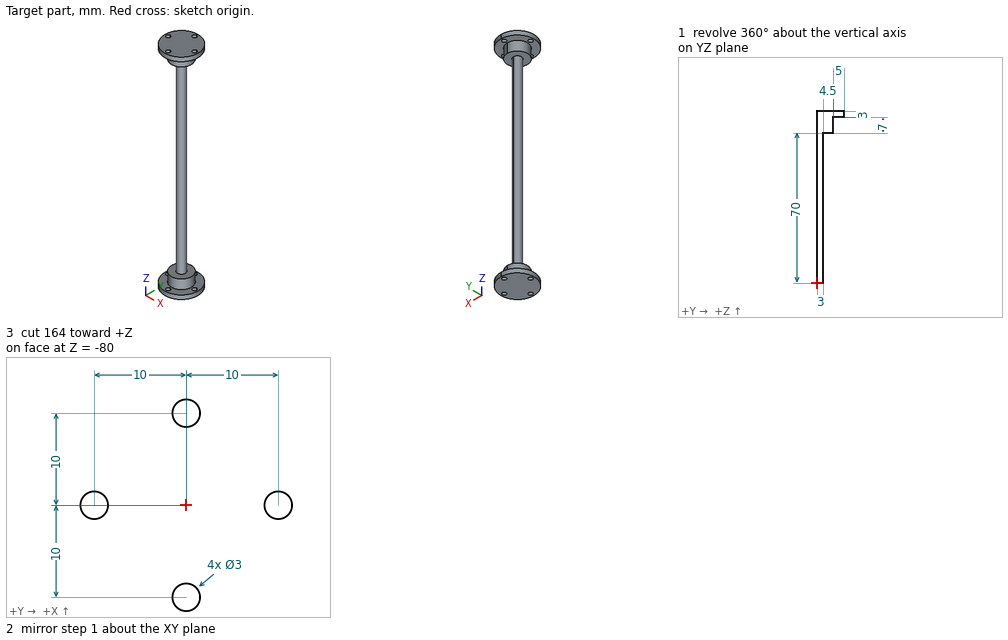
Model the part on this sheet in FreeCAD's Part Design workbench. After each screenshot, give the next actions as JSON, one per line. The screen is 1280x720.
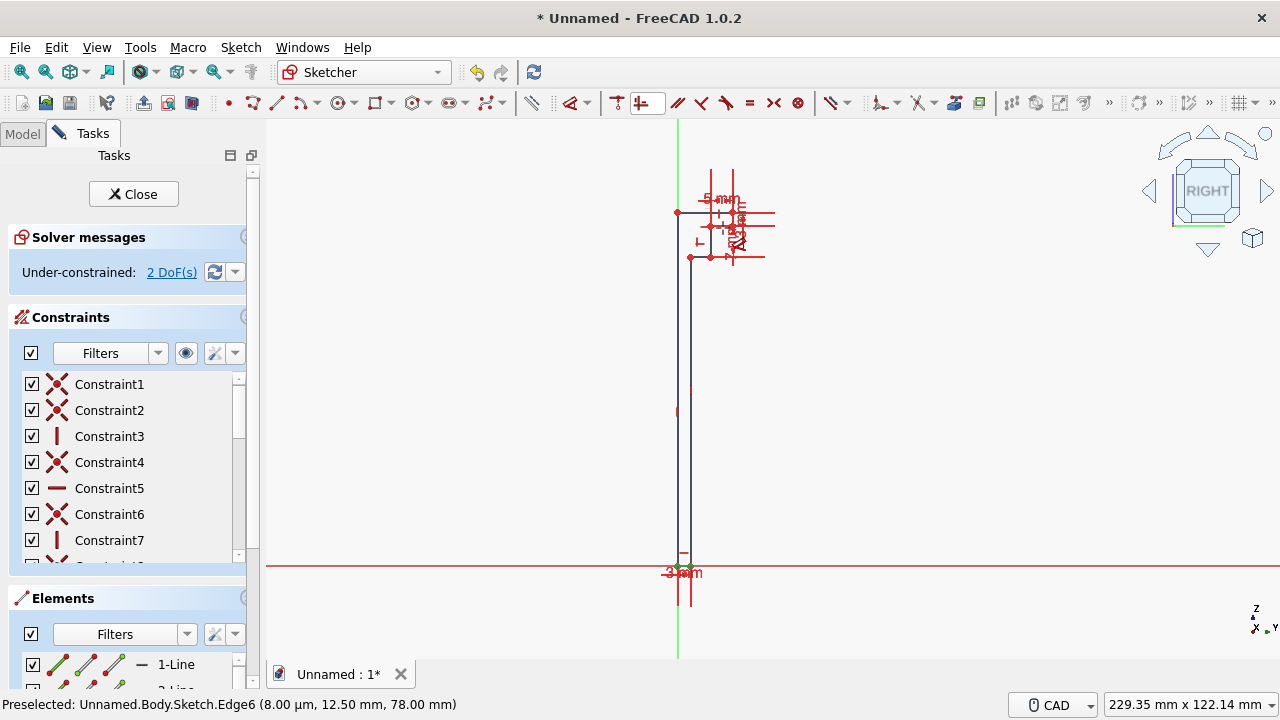
{"action": "left_click", "coordinate": [691, 319]}
{"action": "left_click", "coordinate": [657, 412]}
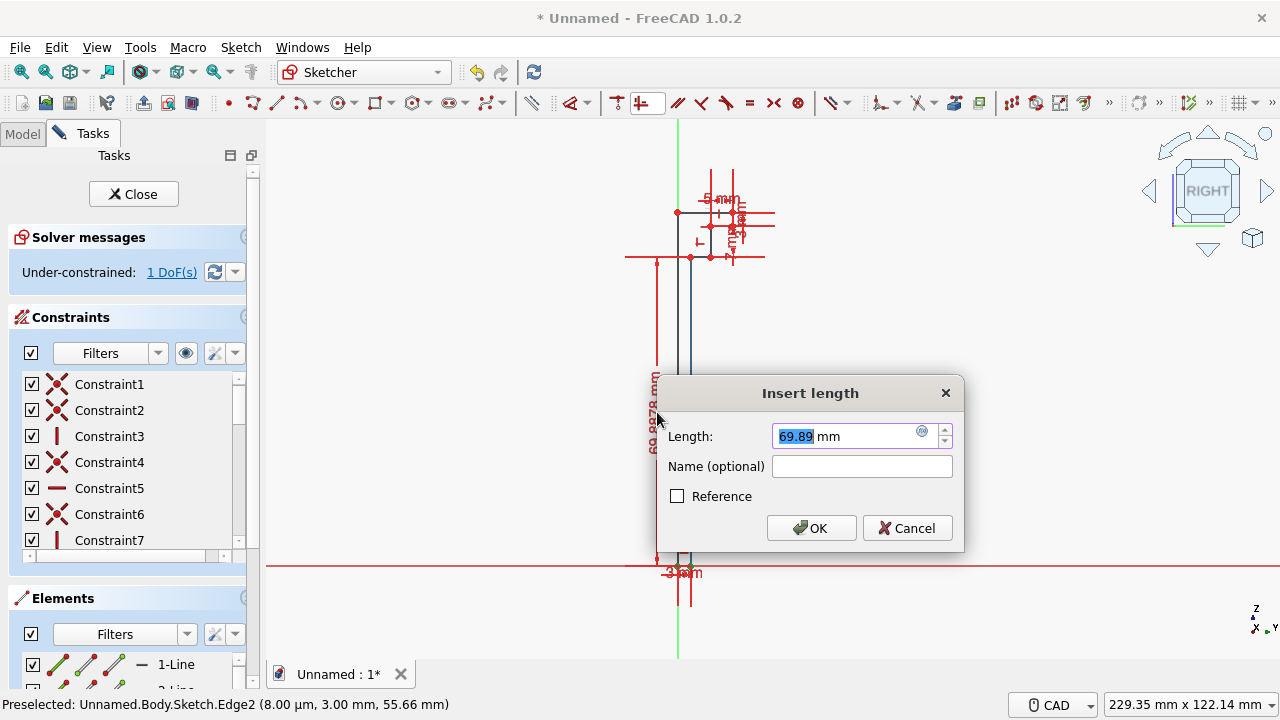
{"action": "type", "text": "70"}
{"action": "key", "text": "Return"}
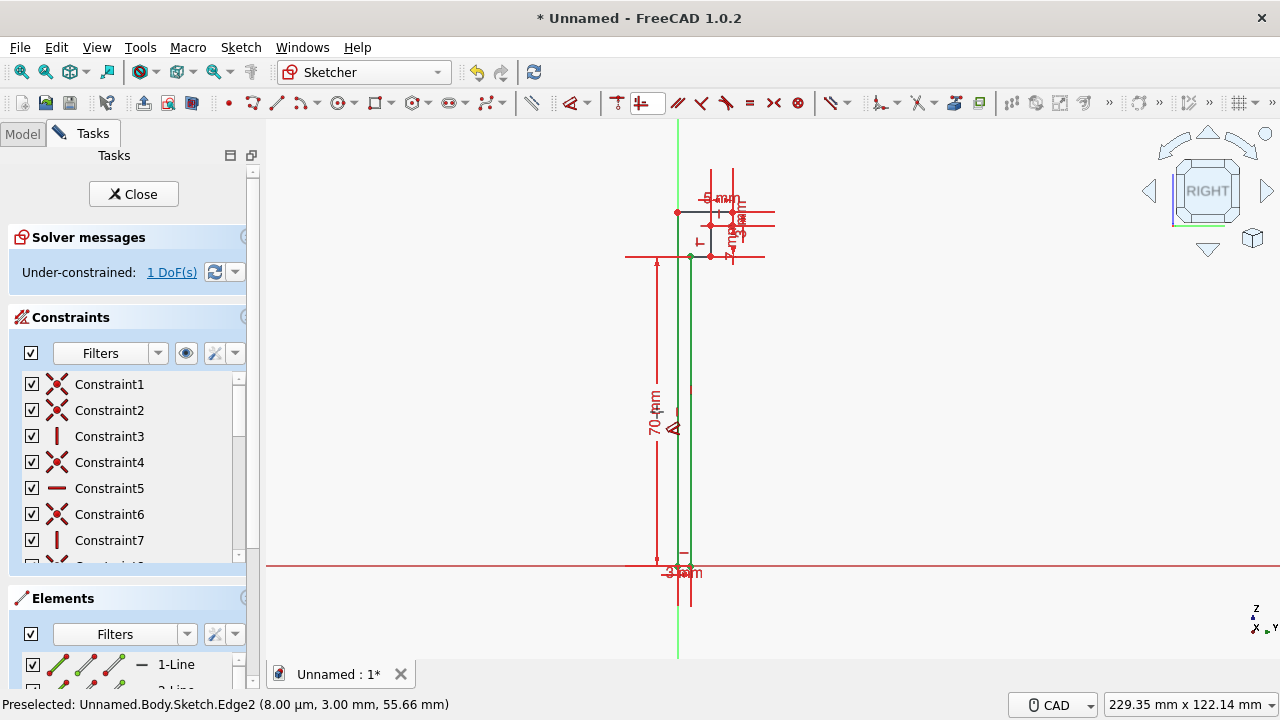
{"action": "scroll", "coordinate": [701, 257], "scroll_direction": "up", "scroll_amount": 4}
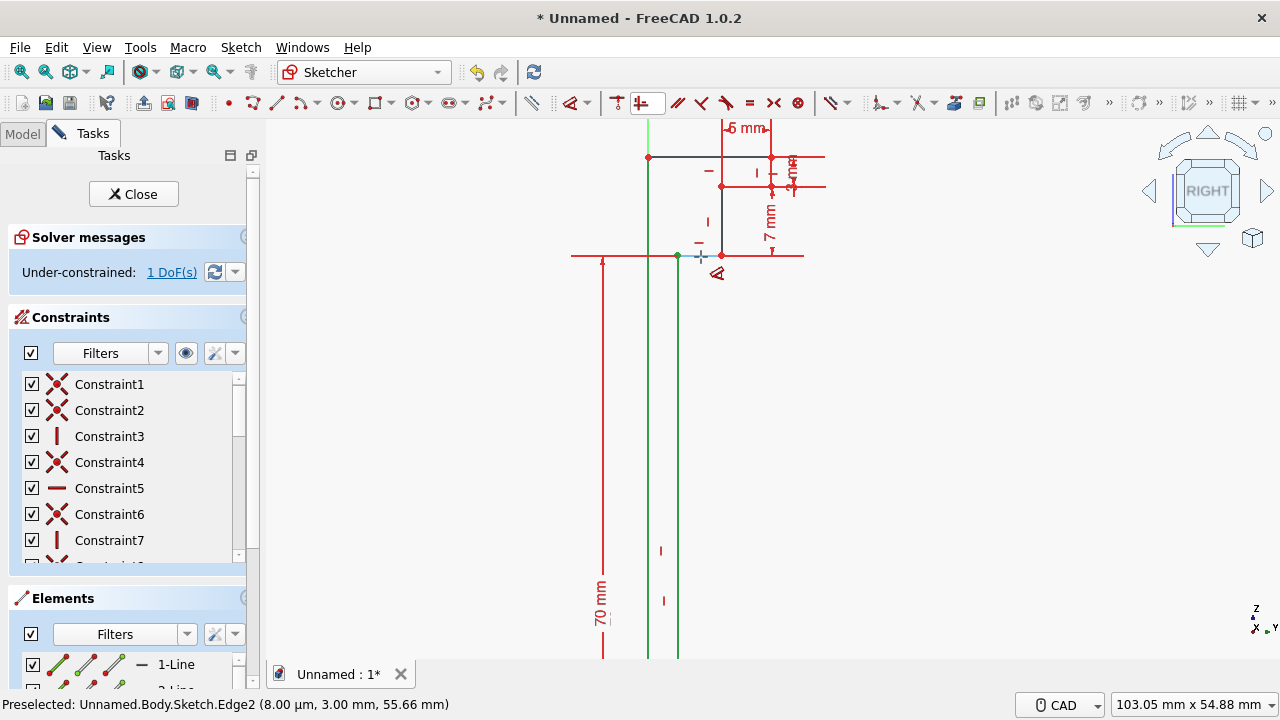
{"action": "left_click", "coordinate": [700, 256]}
{"action": "left_click", "coordinate": [700, 222]}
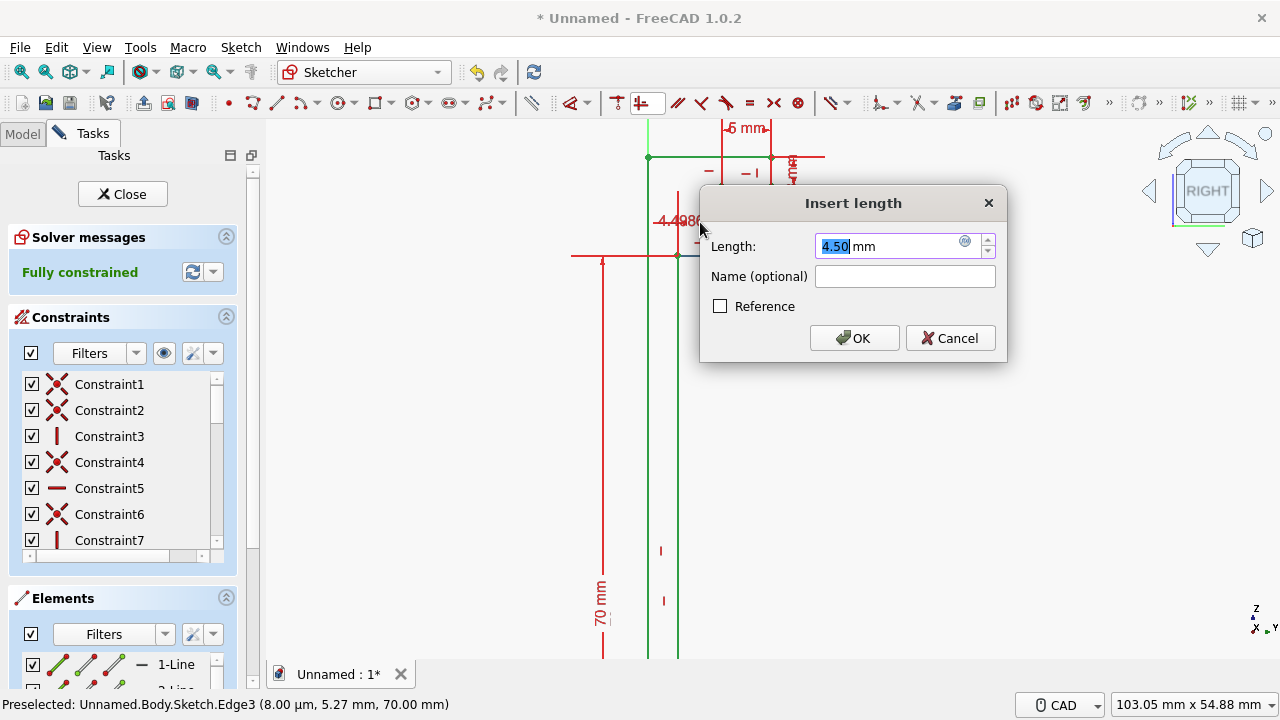
{"action": "type", "text": "4.5"}
{"action": "key", "text": "Return"}
{"action": "key", "text": "Escape"}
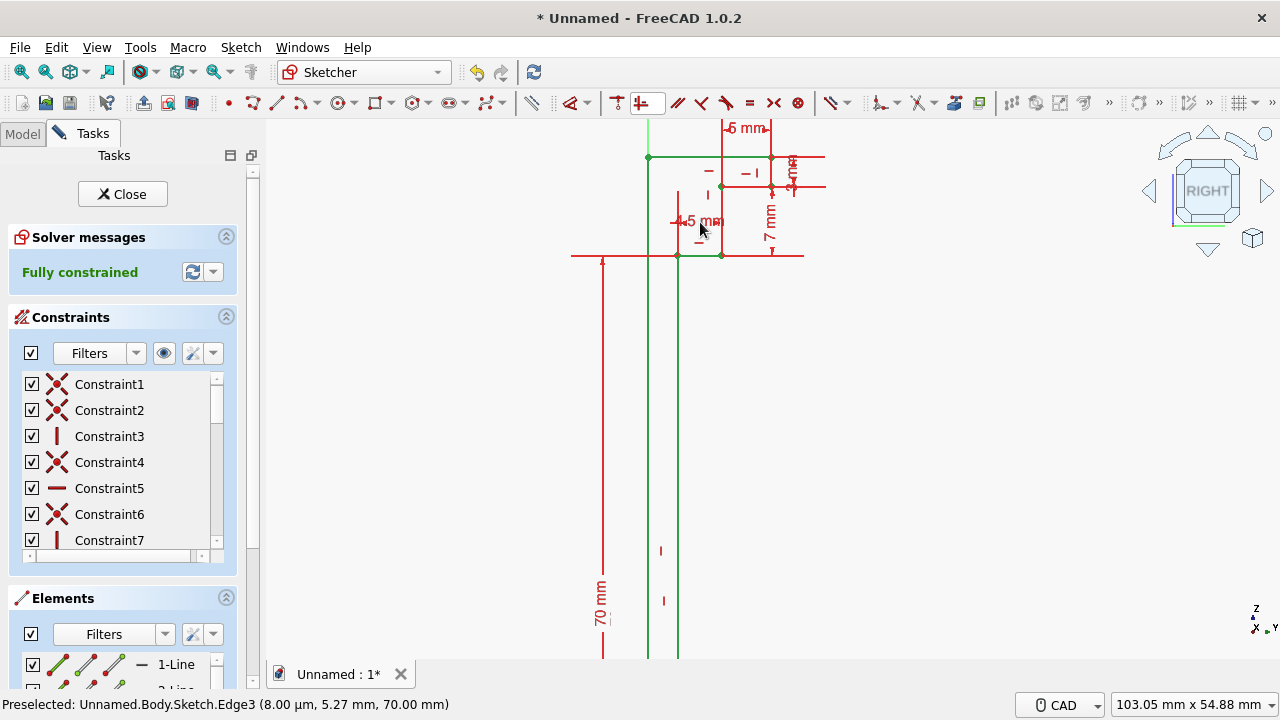
{"action": "left_click", "coordinate": [123, 194]}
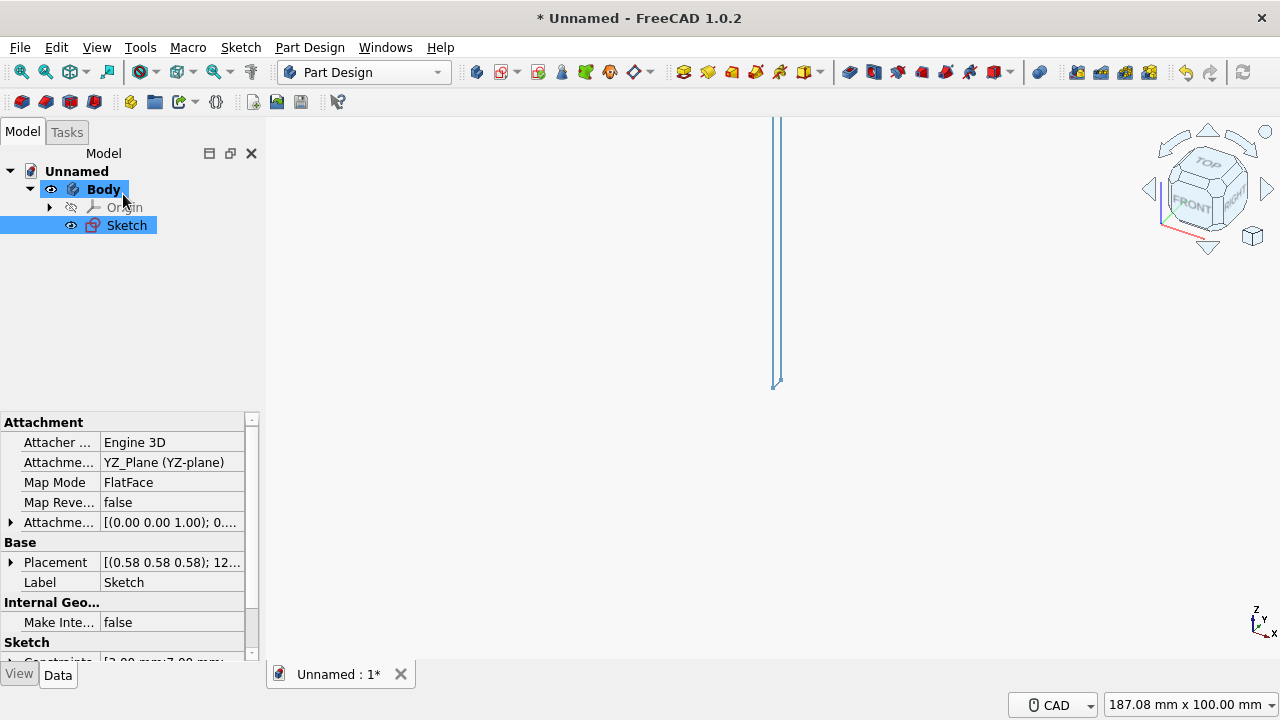
{"action": "left_click", "coordinate": [708, 72]}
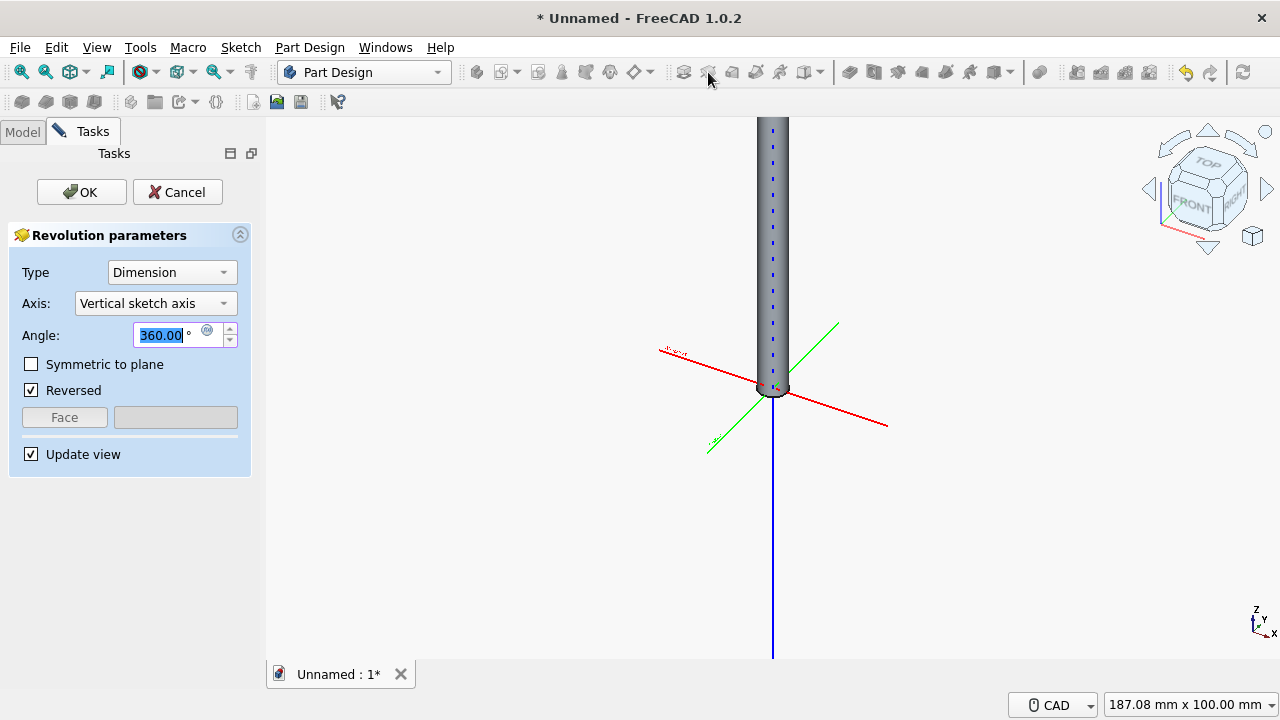
{"action": "left_click", "coordinate": [82, 192]}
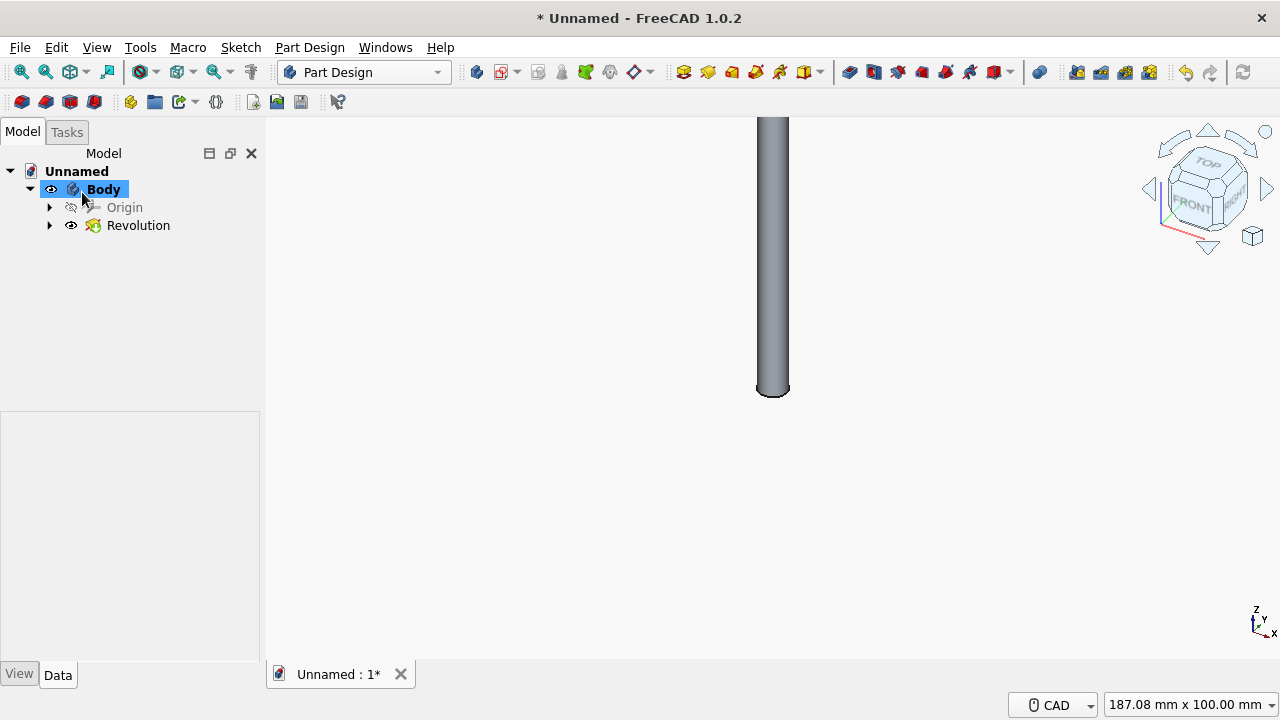
{"action": "left_click", "coordinate": [22, 72]}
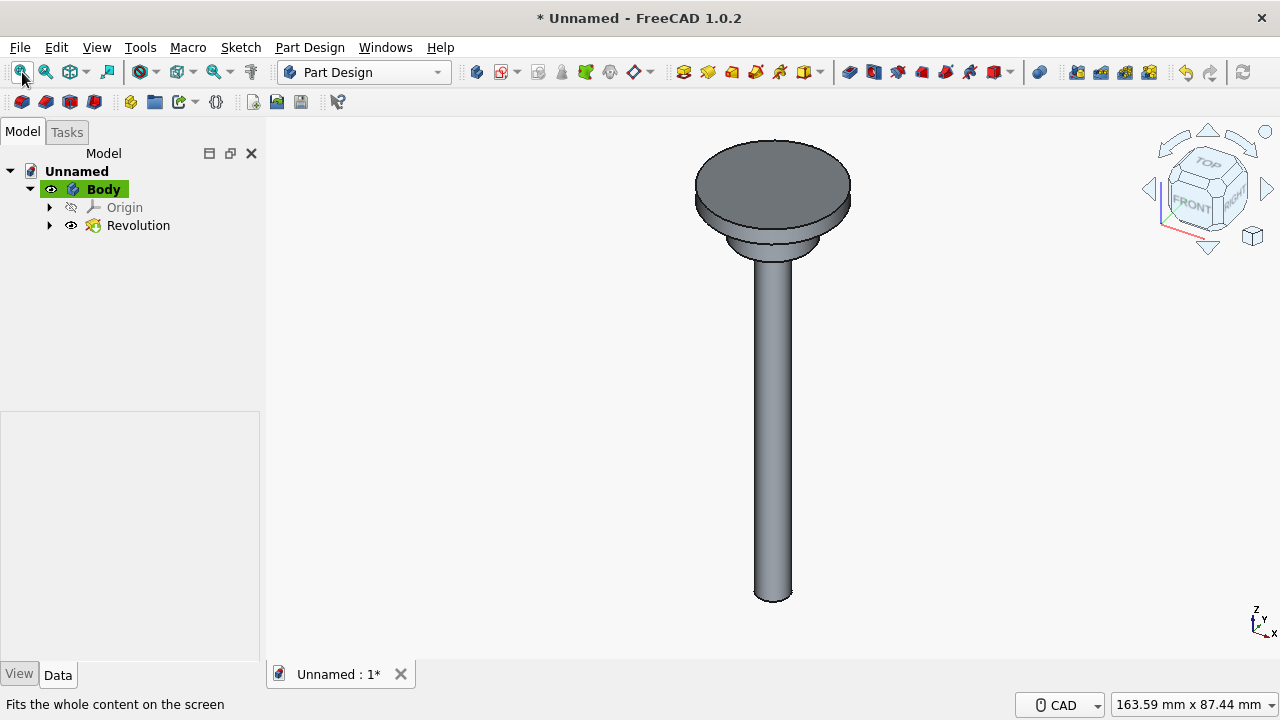
{"action": "left_click", "coordinate": [116, 225]}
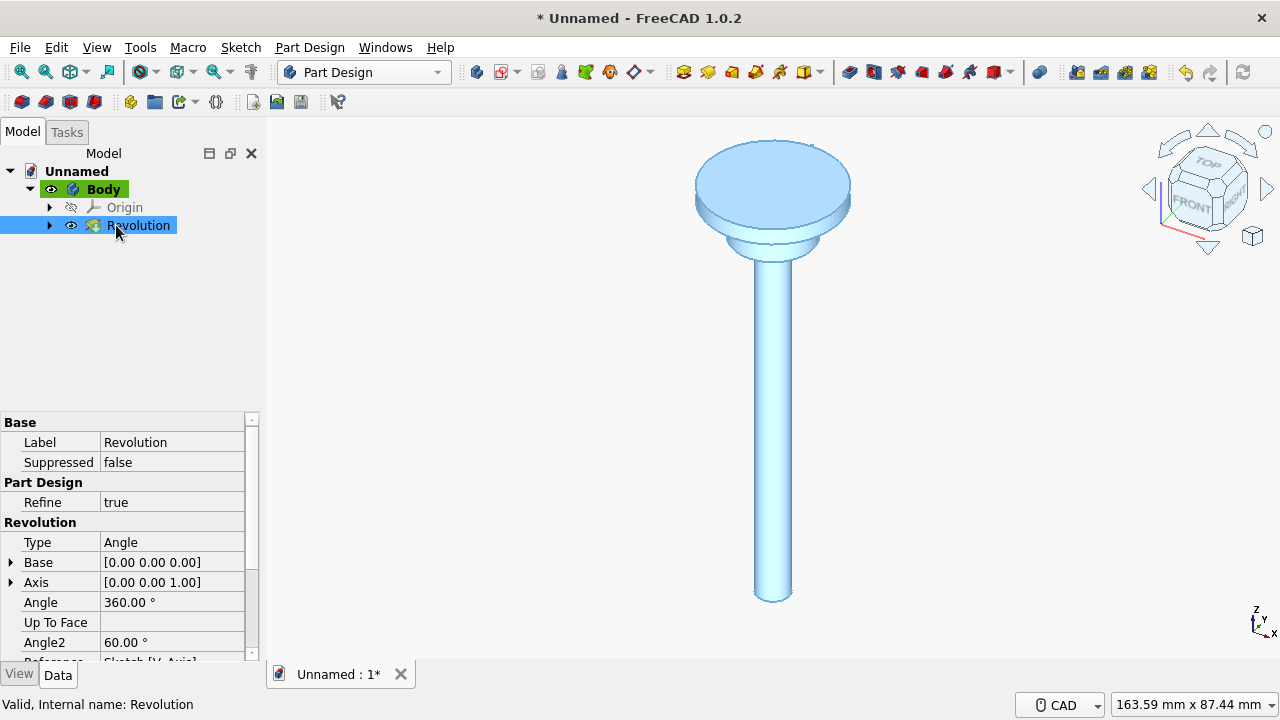
{"action": "left_click", "coordinate": [1078, 72]}